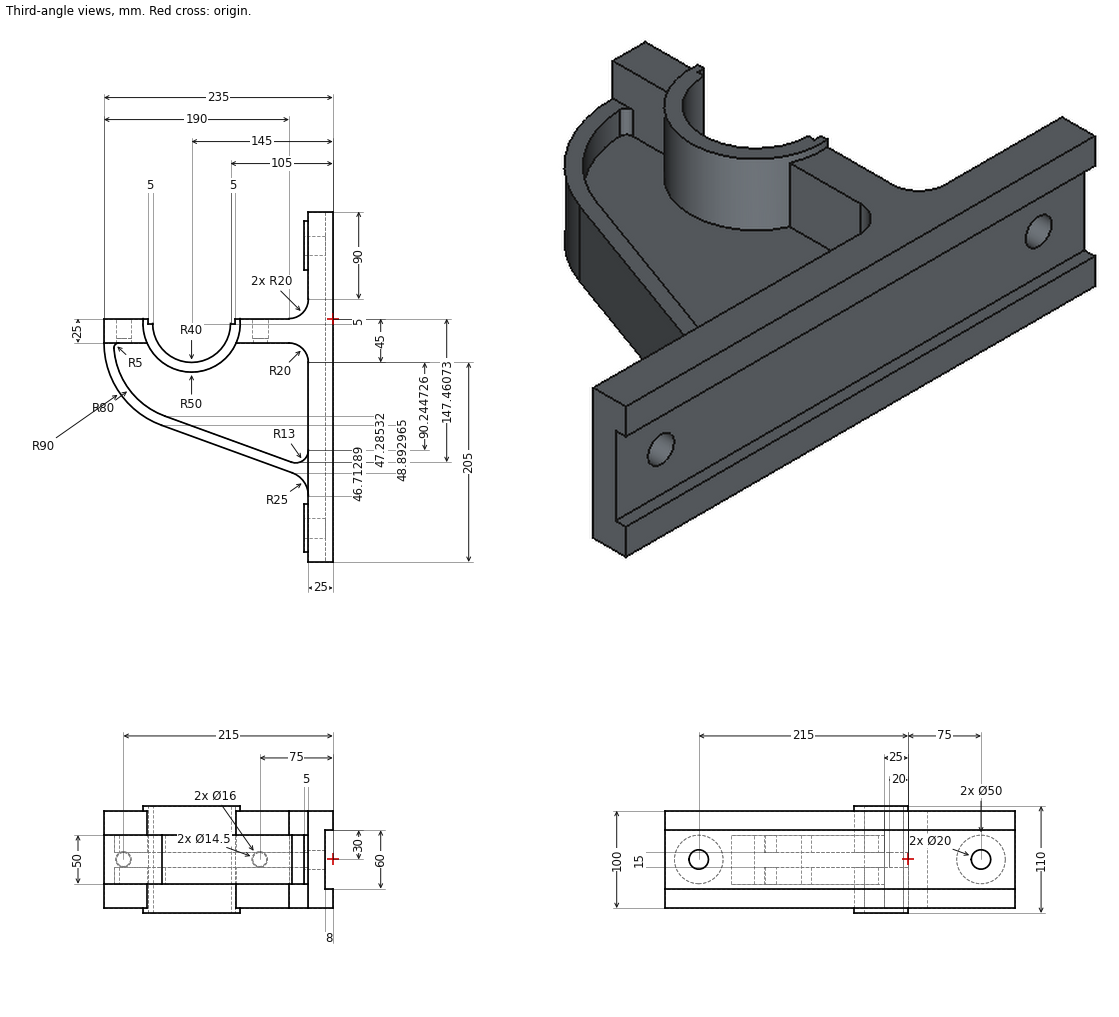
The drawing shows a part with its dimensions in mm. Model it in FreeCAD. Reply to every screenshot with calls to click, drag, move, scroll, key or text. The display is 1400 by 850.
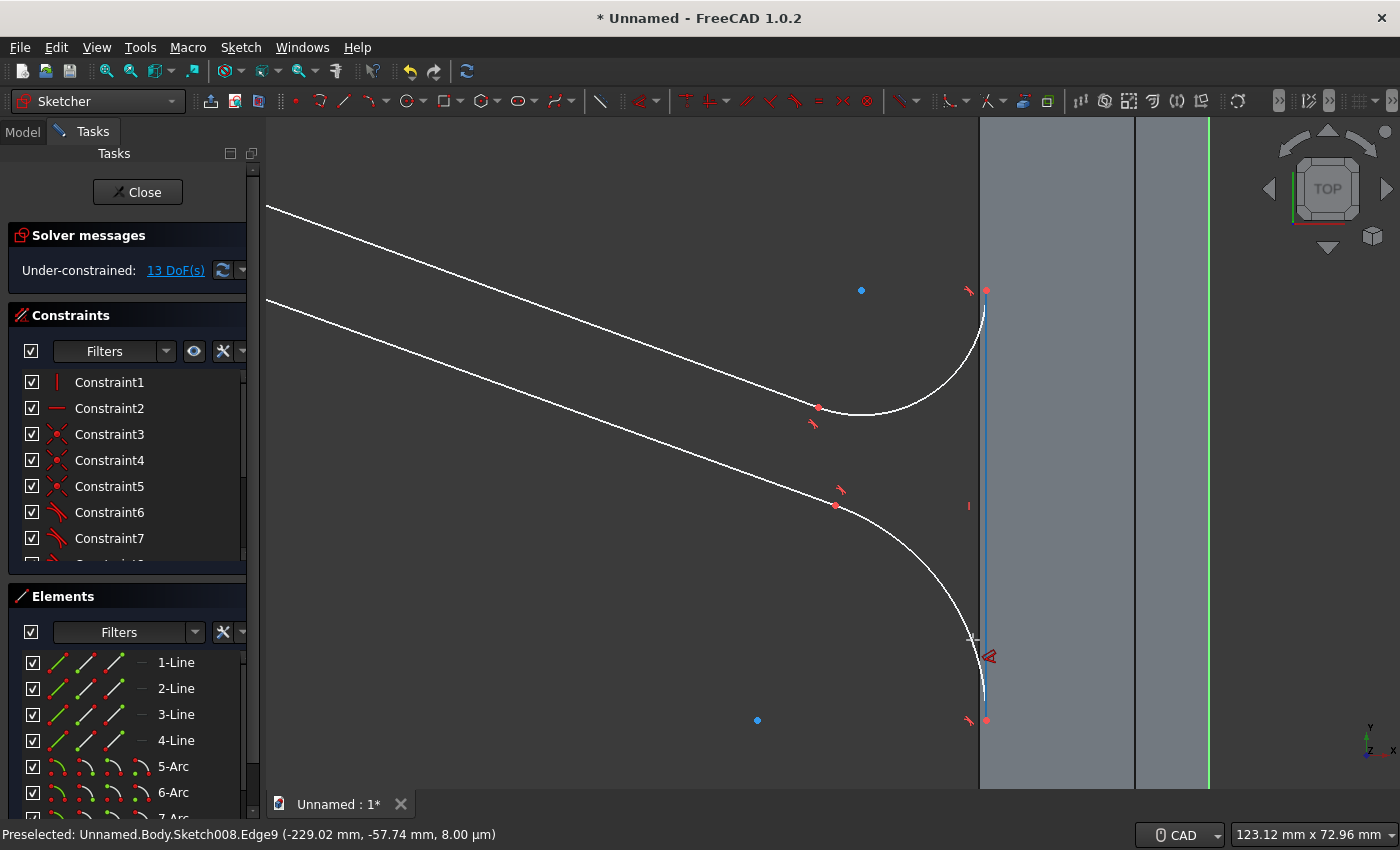
click(971, 638)
click(1001, 626)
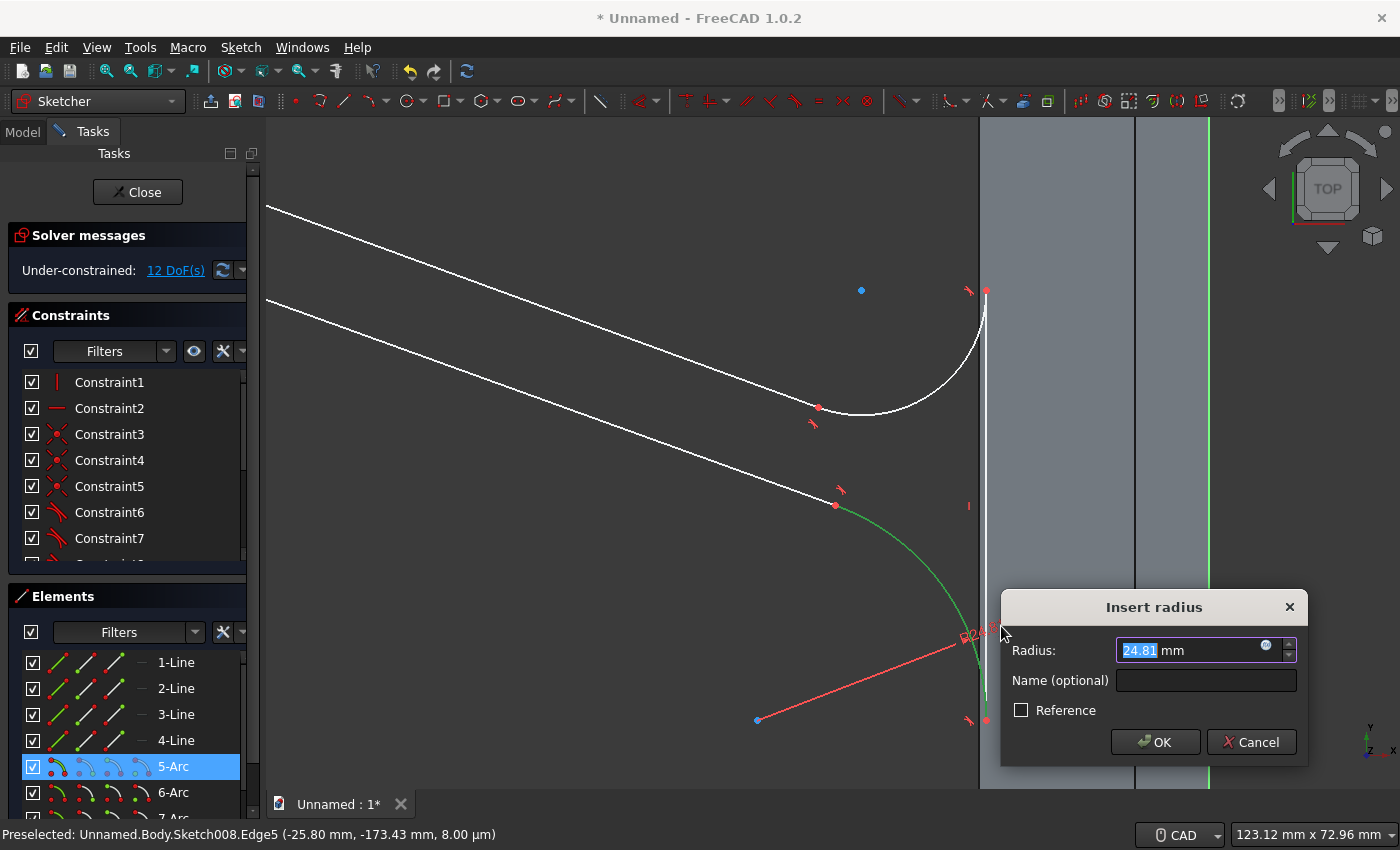
text(25)
key(Return)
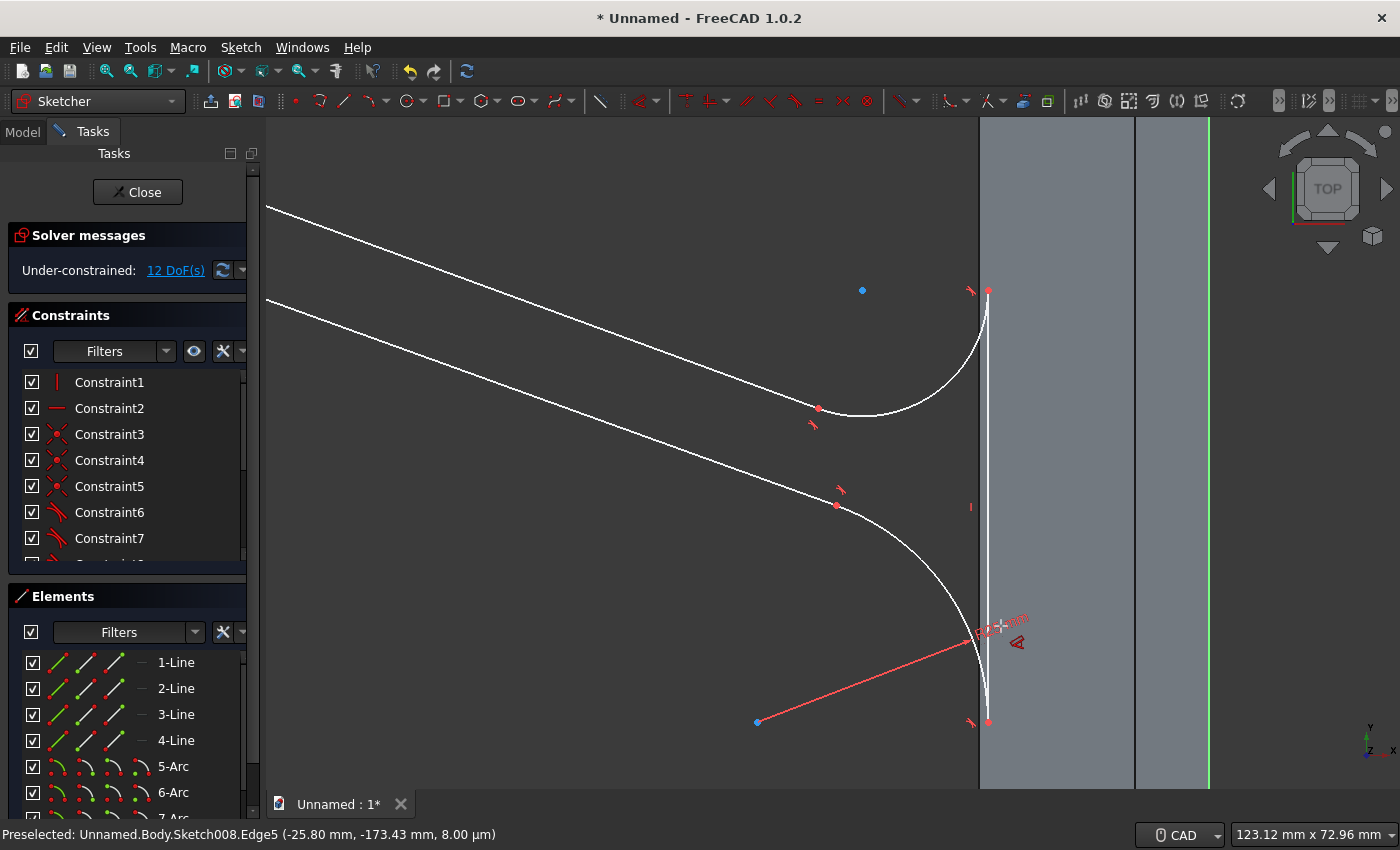
scroll(973, 641, down, 7)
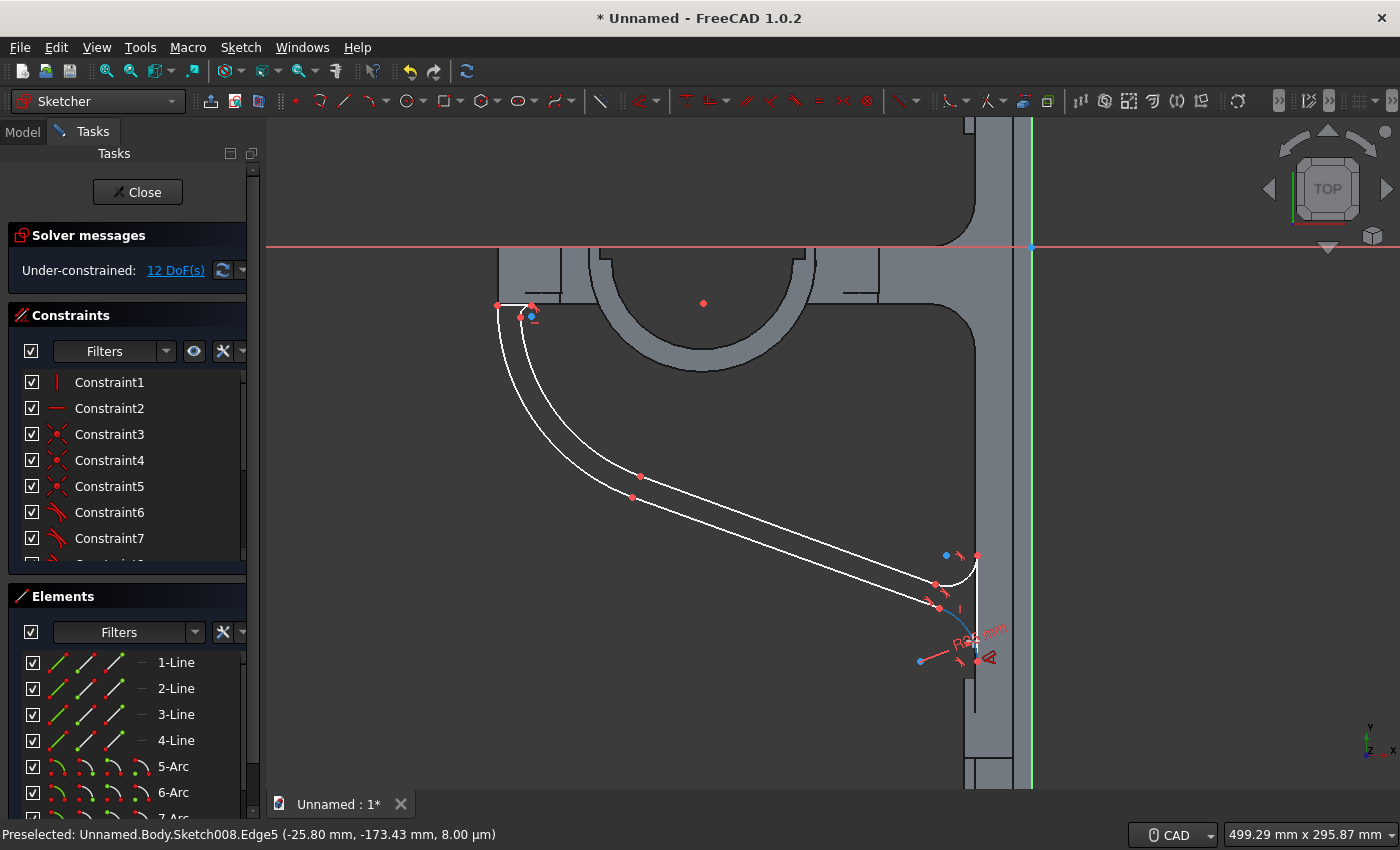
scroll(953, 585, up, 2)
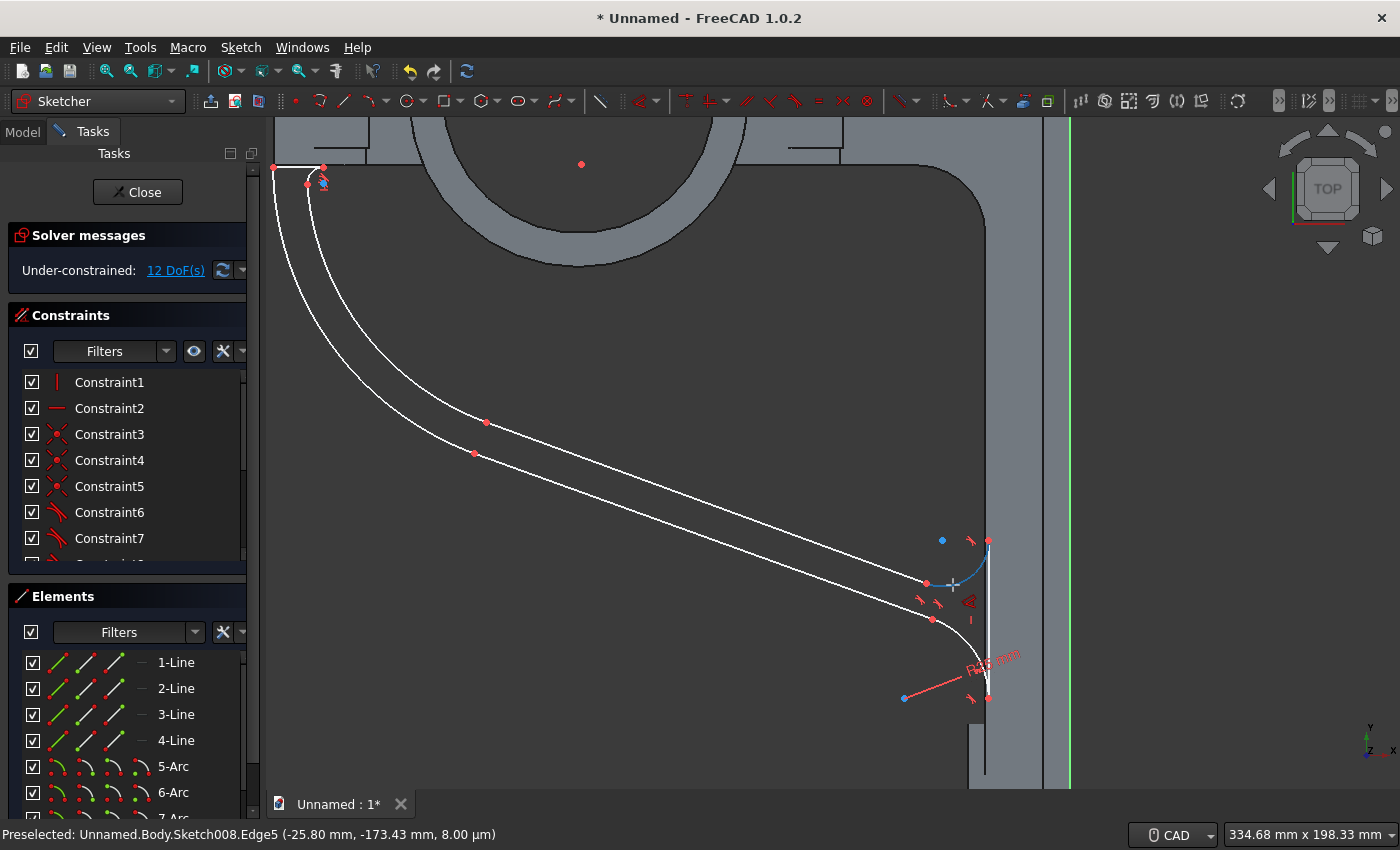
click(953, 585)
click(960, 616)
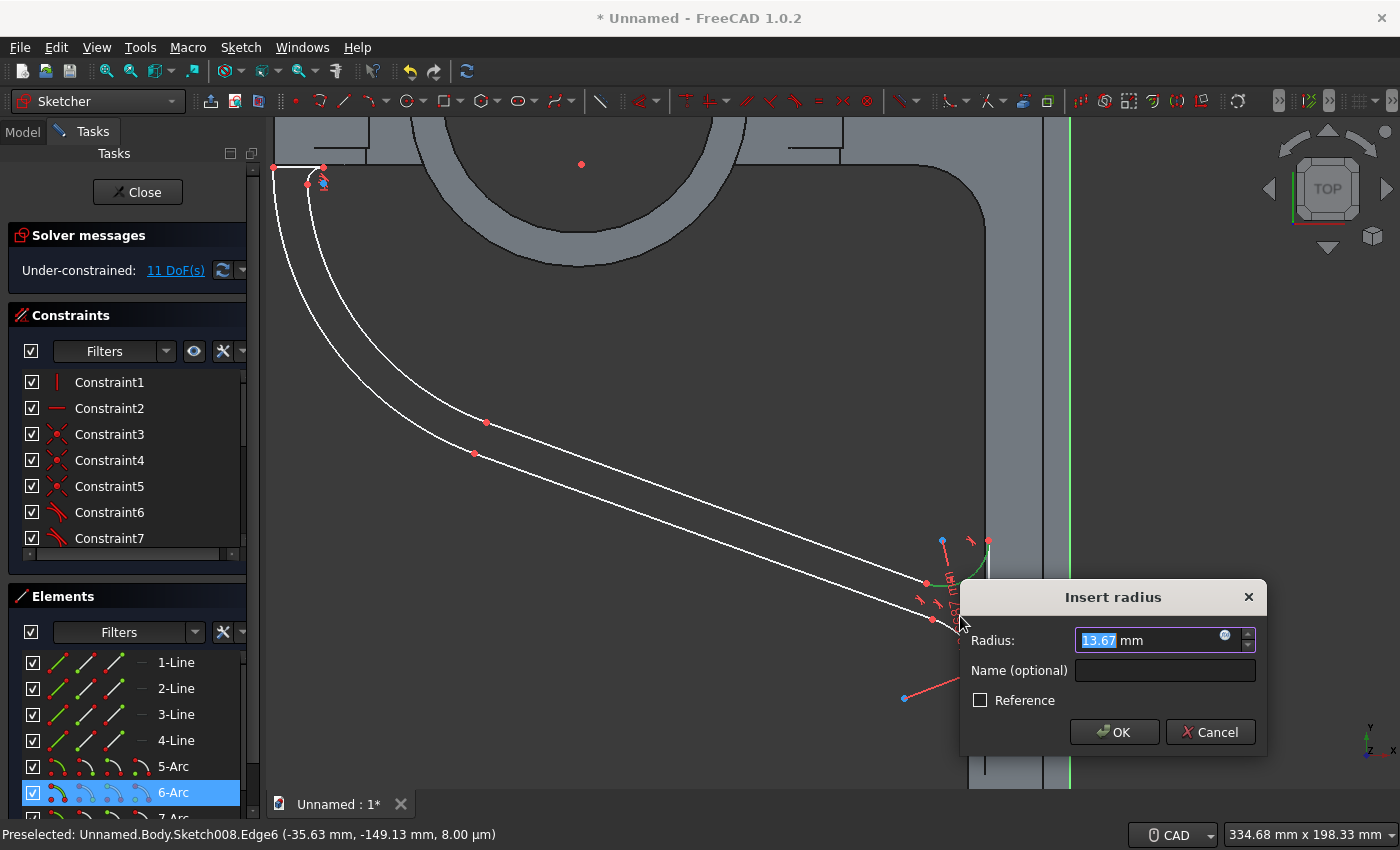
text(13)
key(Return)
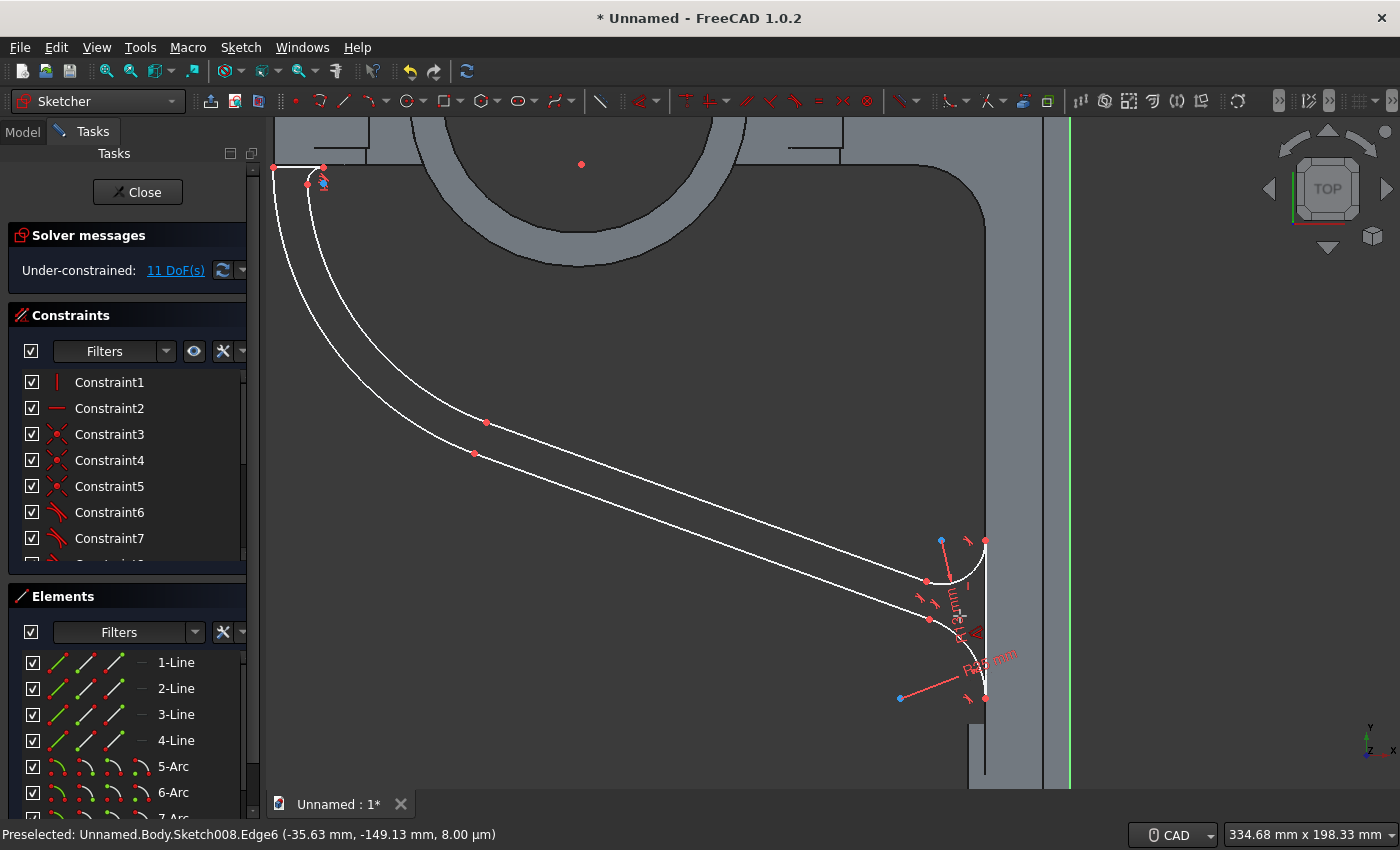
click(330, 276)
click(705, 445)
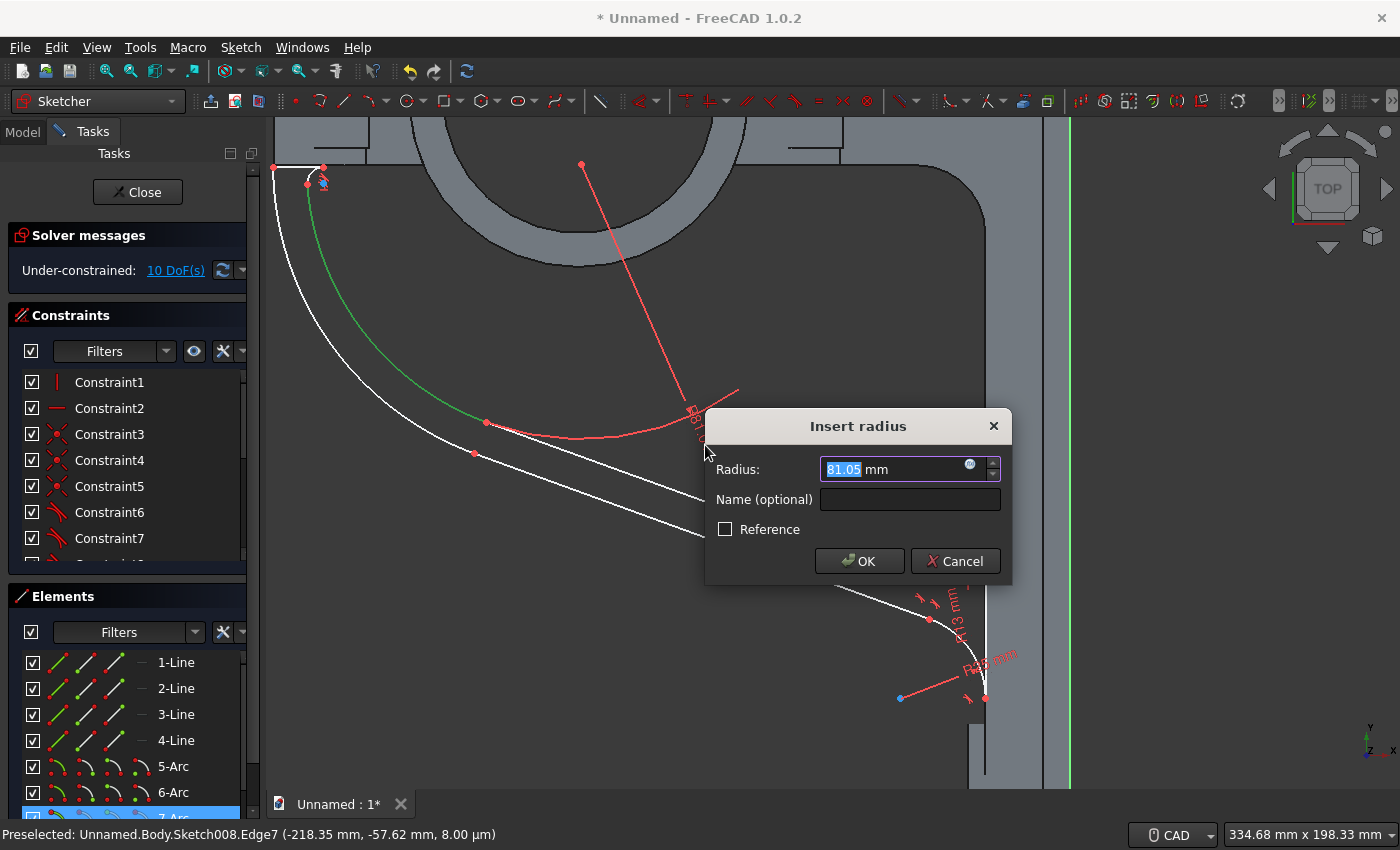
text(80)
key(Return)